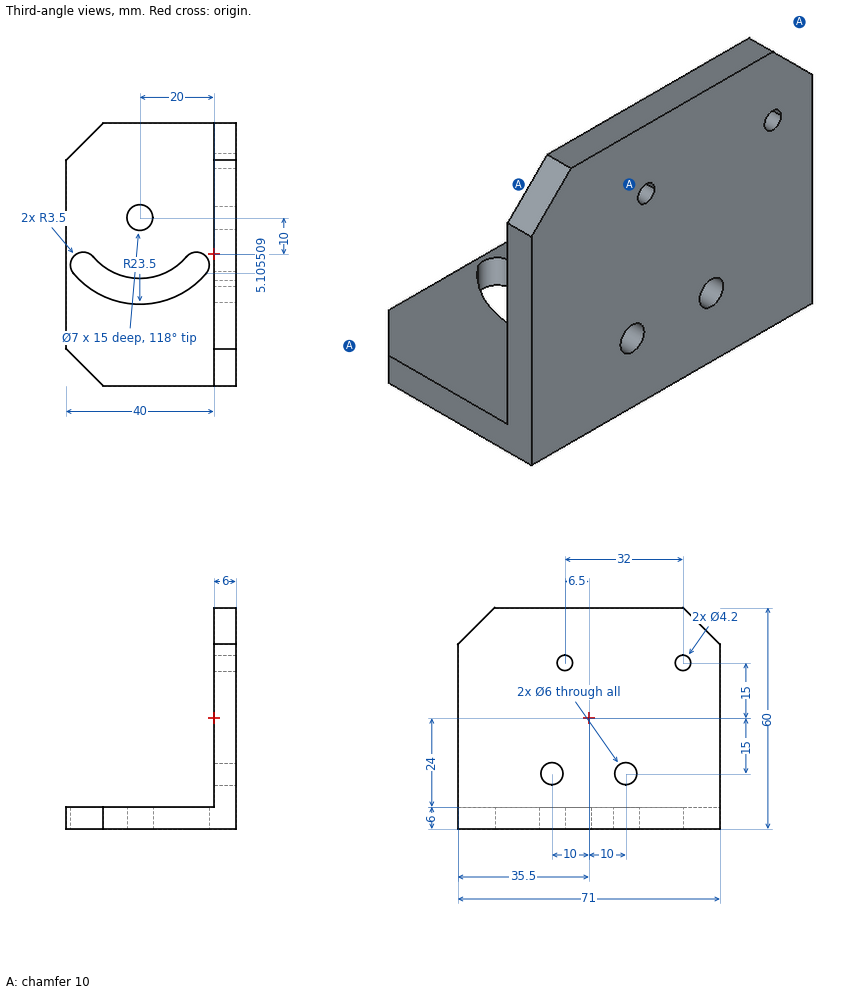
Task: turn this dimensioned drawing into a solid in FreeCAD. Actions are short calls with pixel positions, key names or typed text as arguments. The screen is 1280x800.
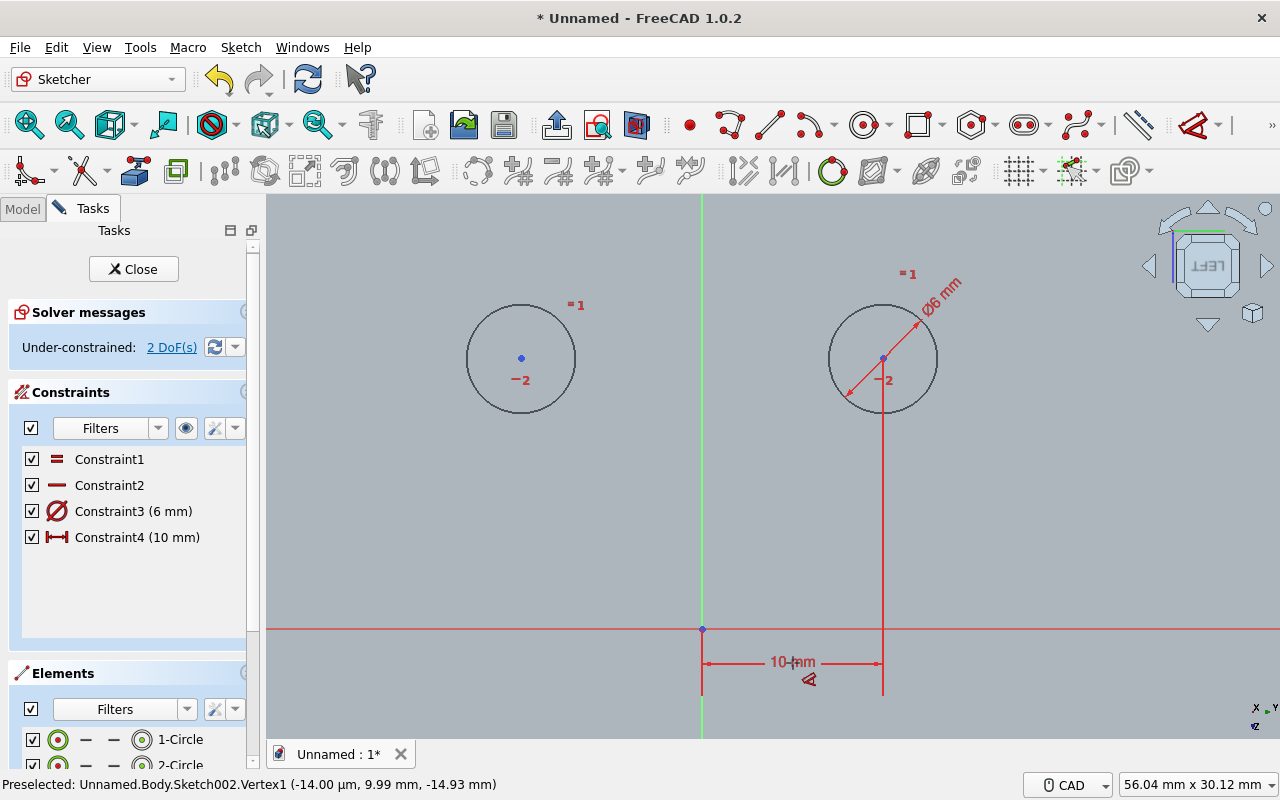
click(883, 359)
click(917, 494)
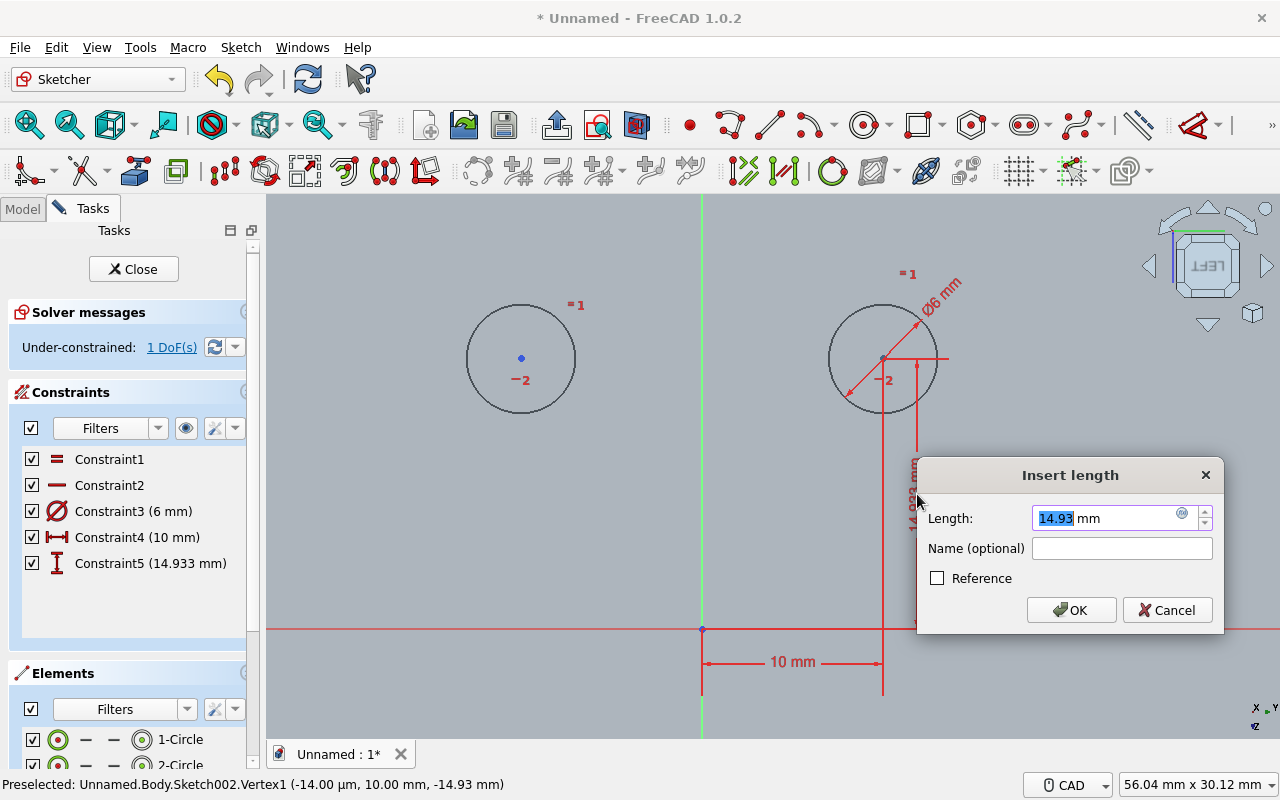
text(15)
key(Return)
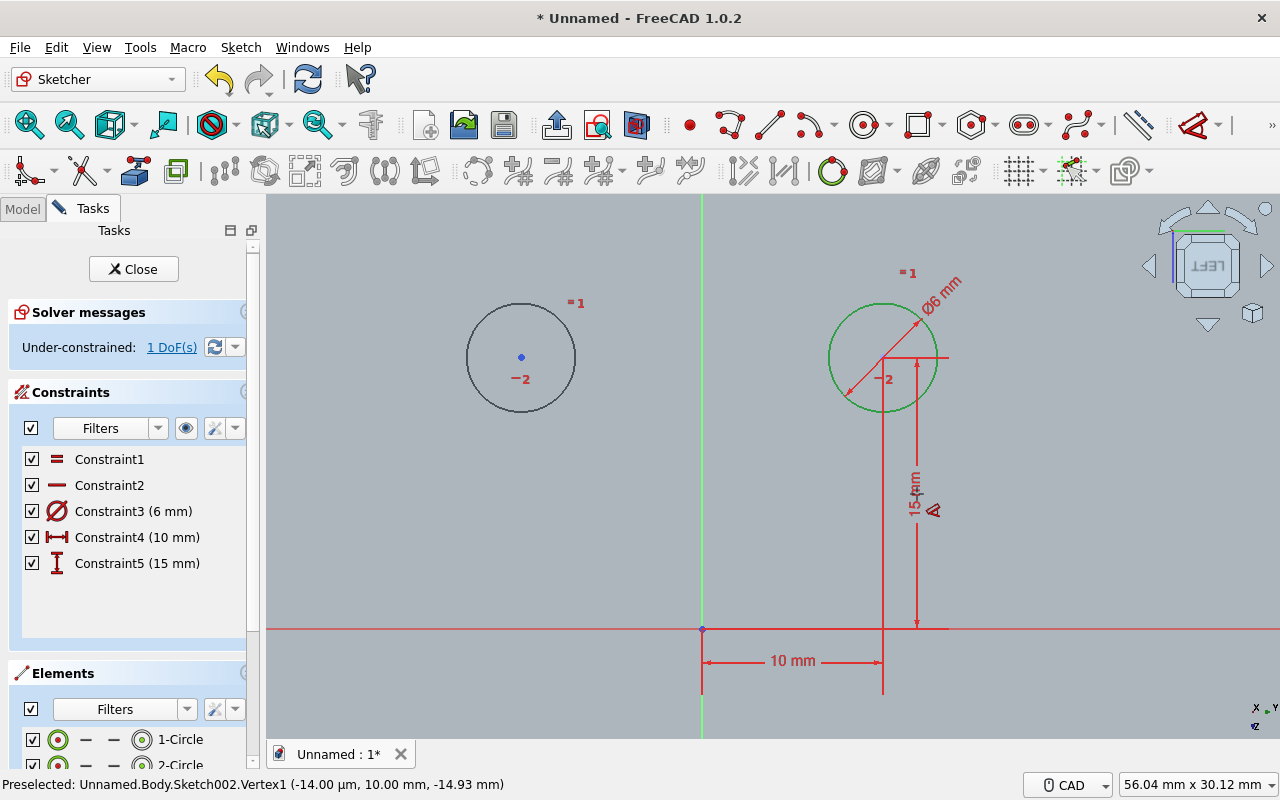
click(521, 358)
click(612, 663)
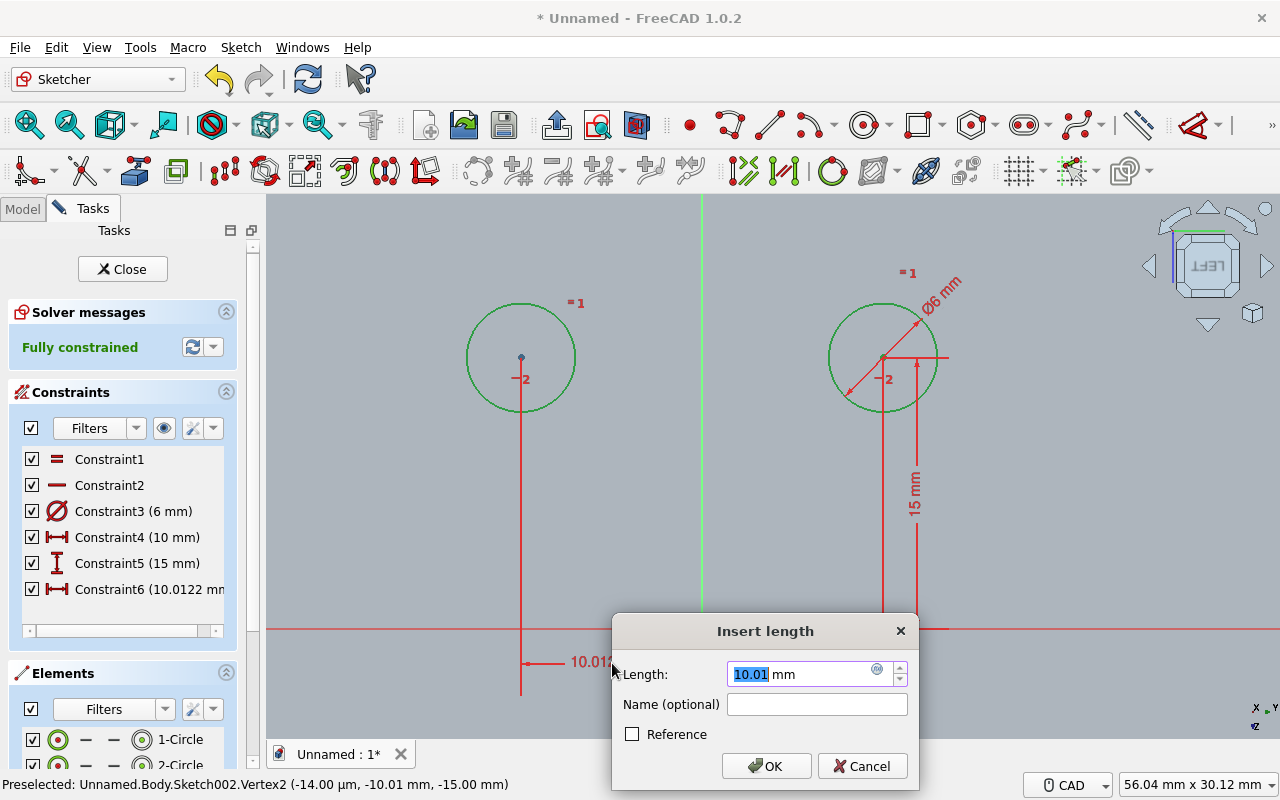
text(10)
key(Return)
key(Escape)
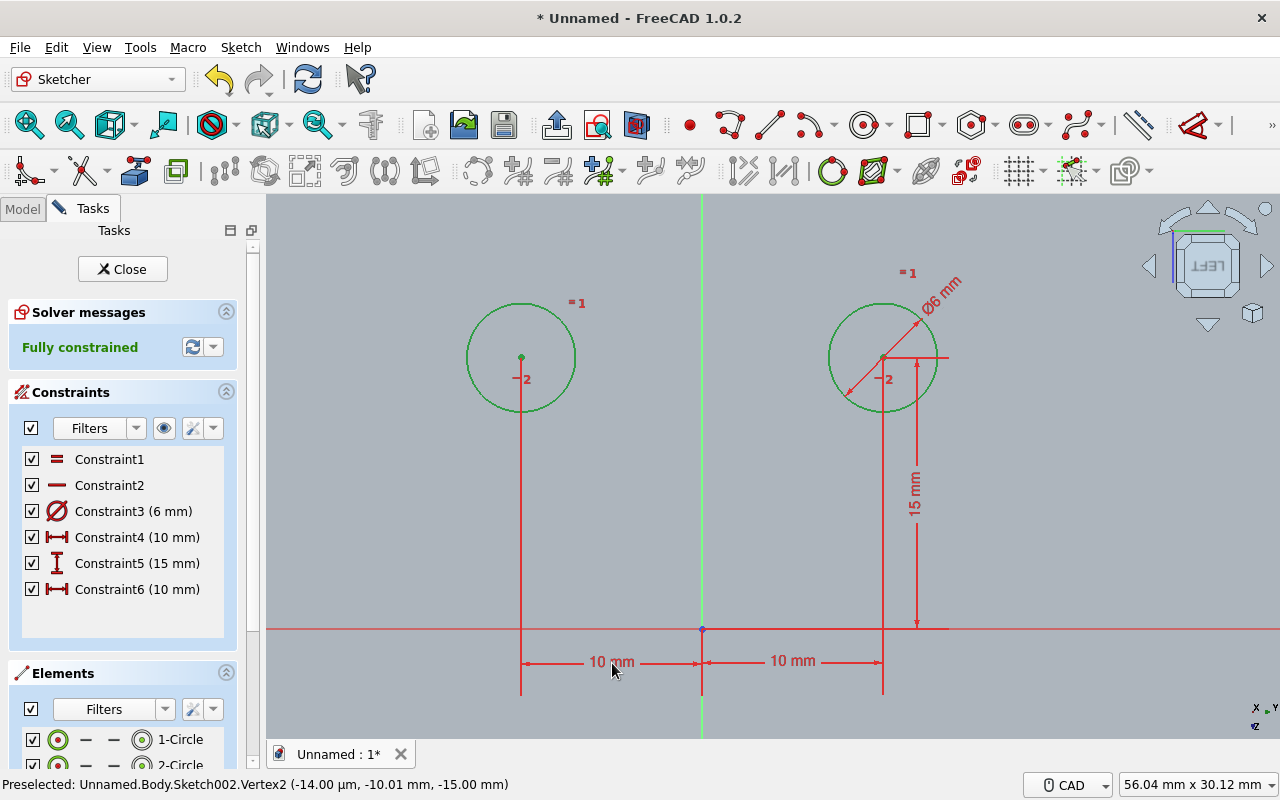
click(123, 269)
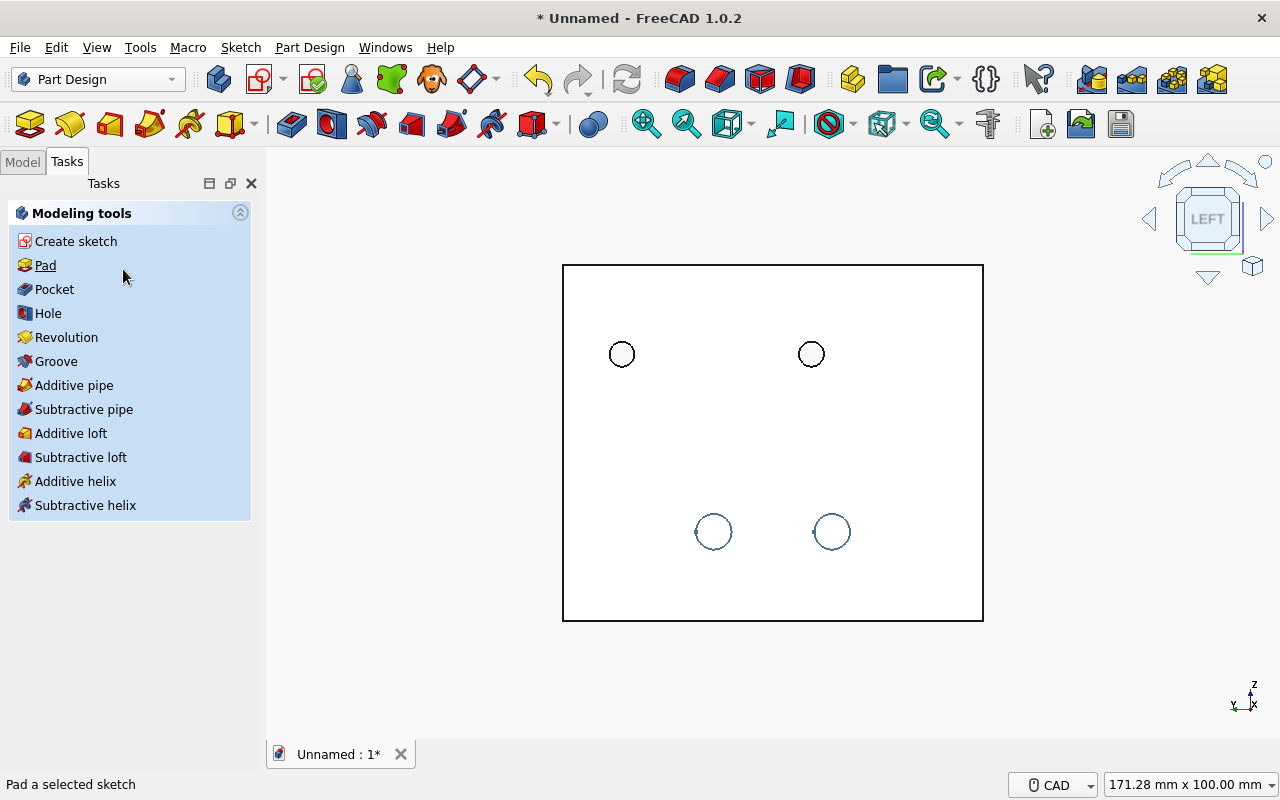
click(332, 124)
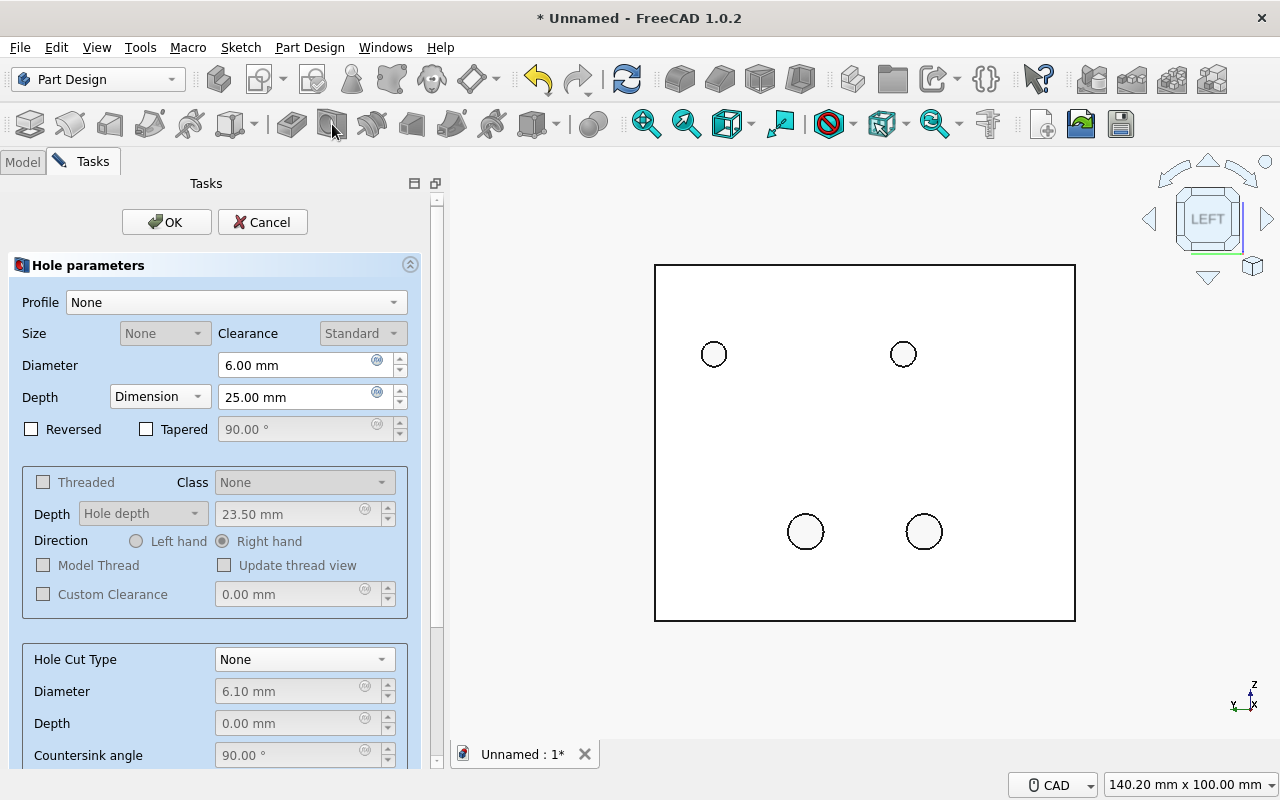
triple_click(305, 365)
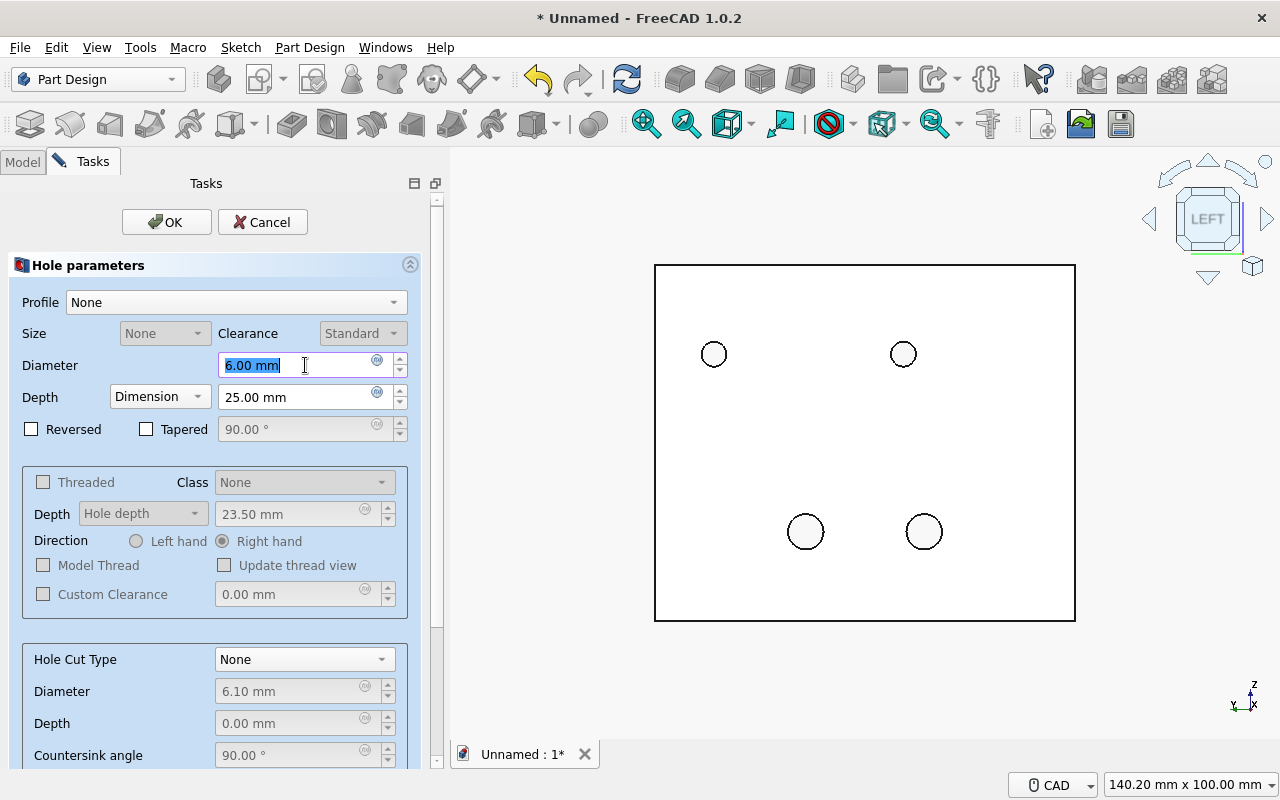
text(6)
key(Tab)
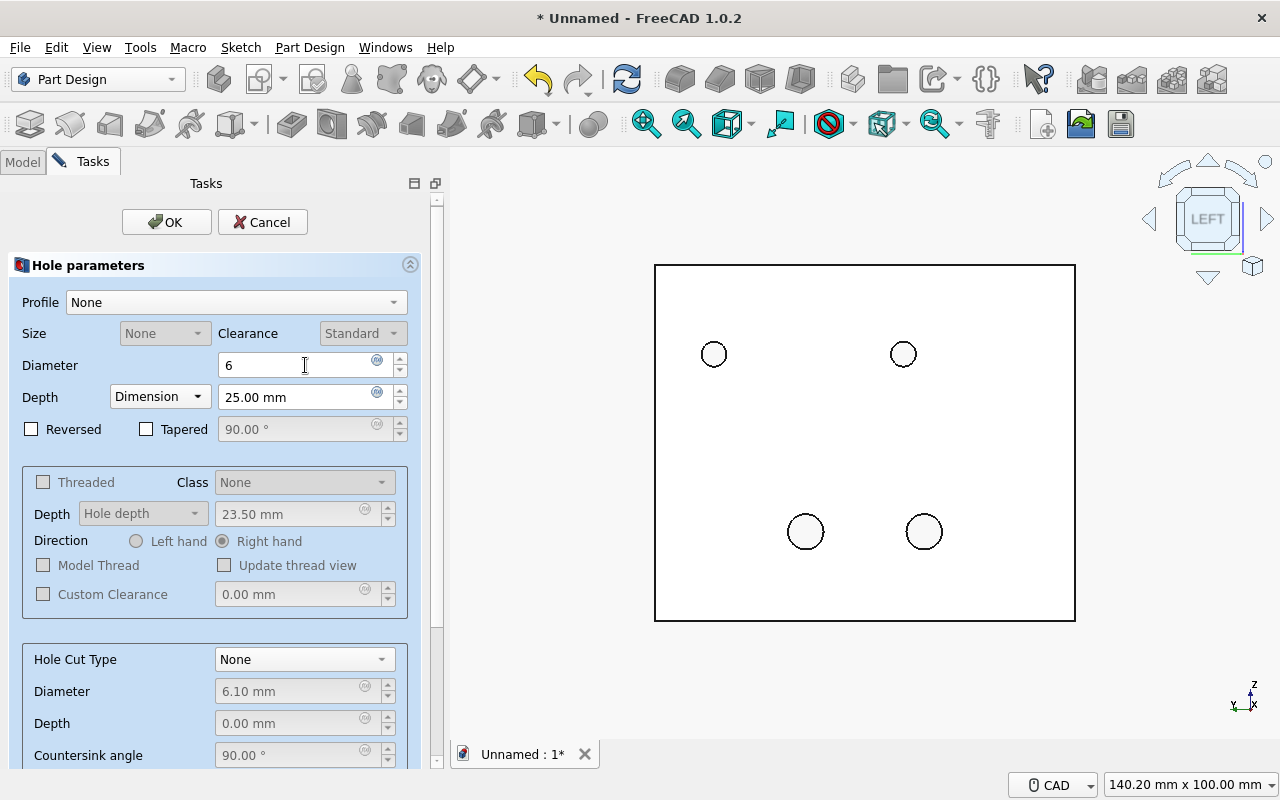
click(161, 396)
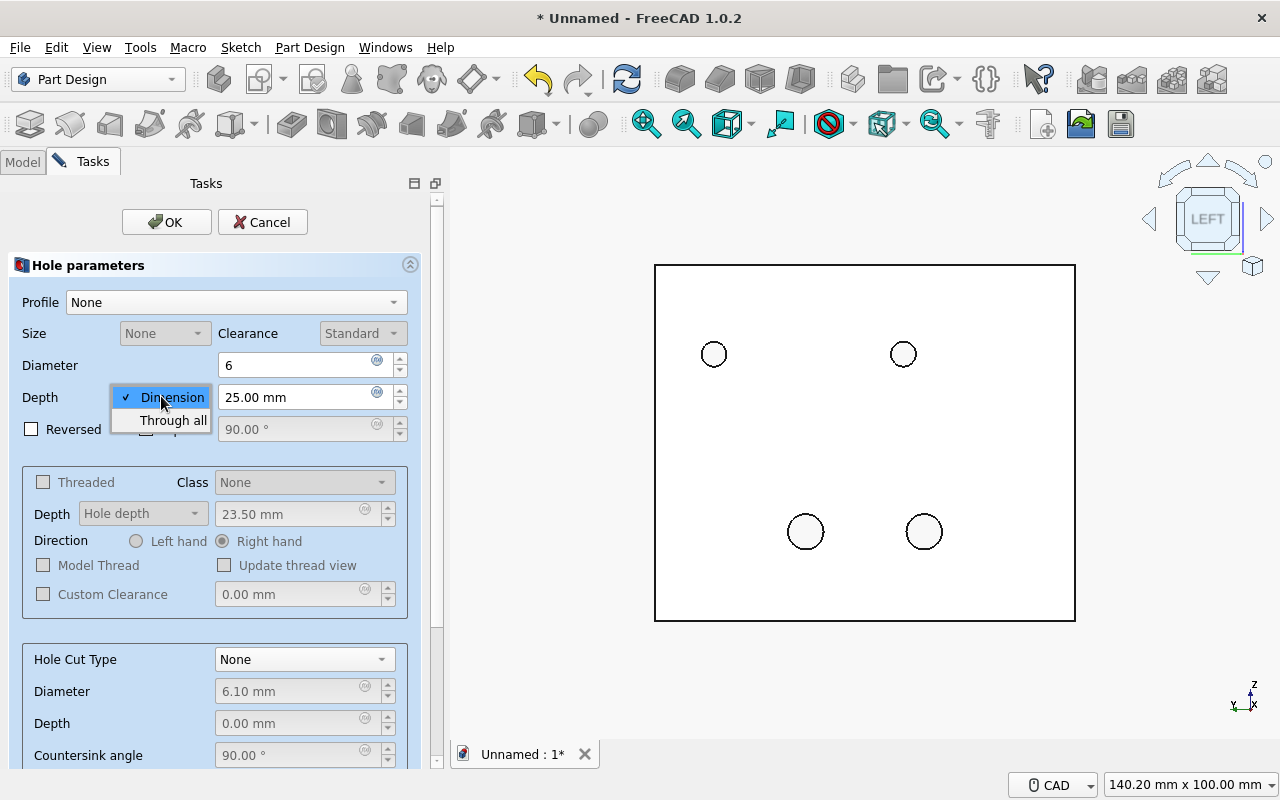
click(160, 420)